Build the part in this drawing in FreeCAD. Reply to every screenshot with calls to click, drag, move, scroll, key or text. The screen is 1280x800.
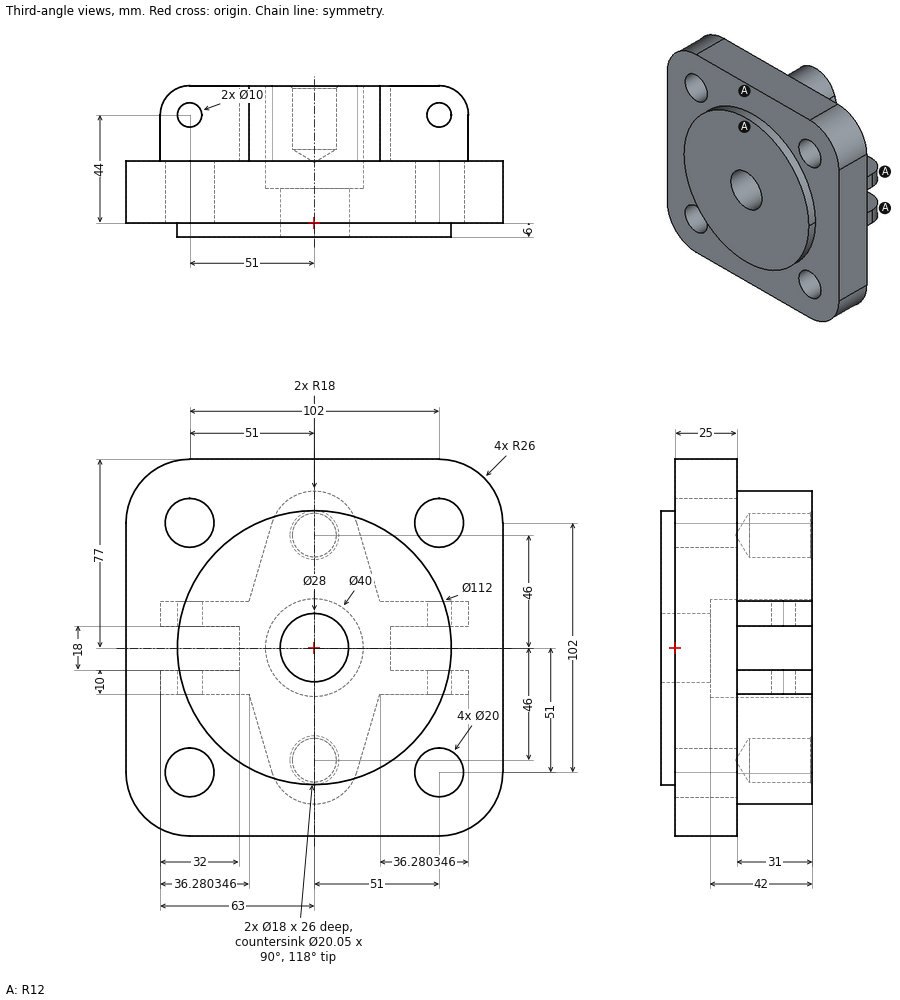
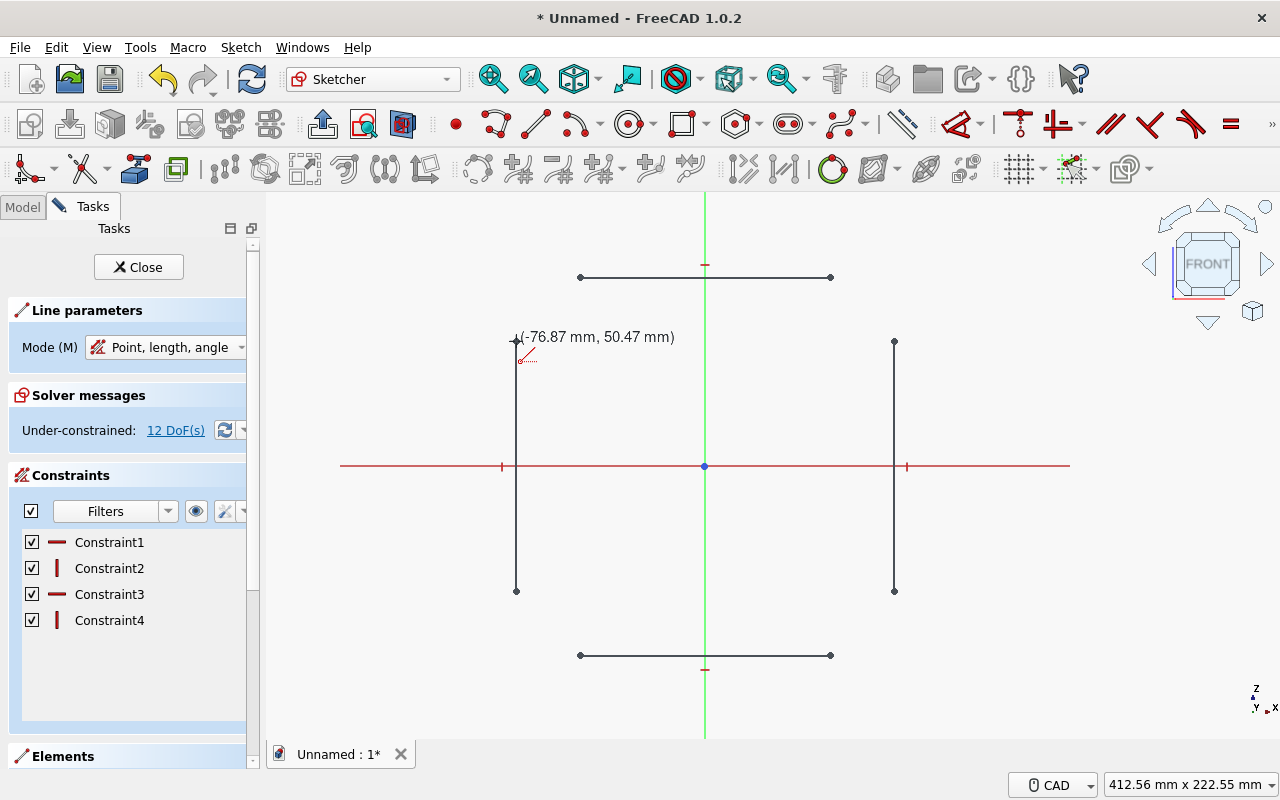
key(g)
key(3)
key(a)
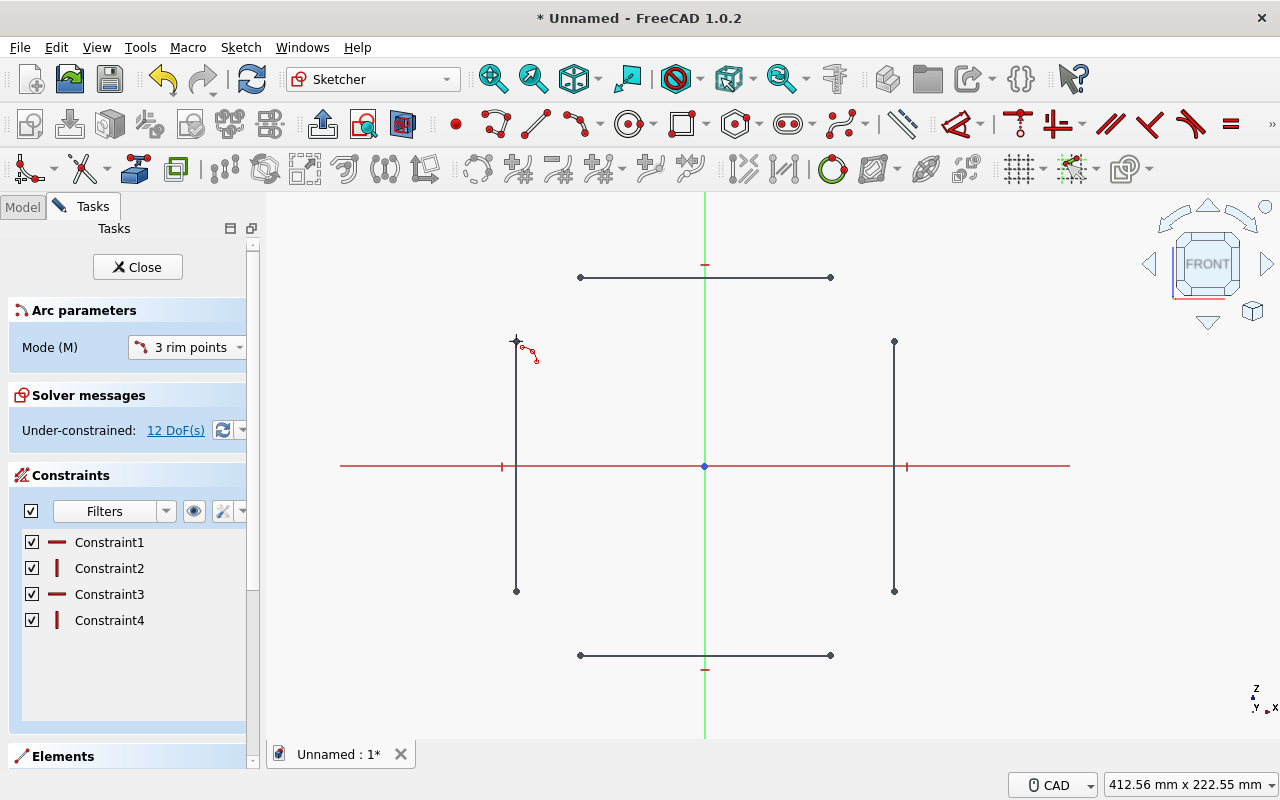
click(830, 278)
click(894, 342)
click(875, 296)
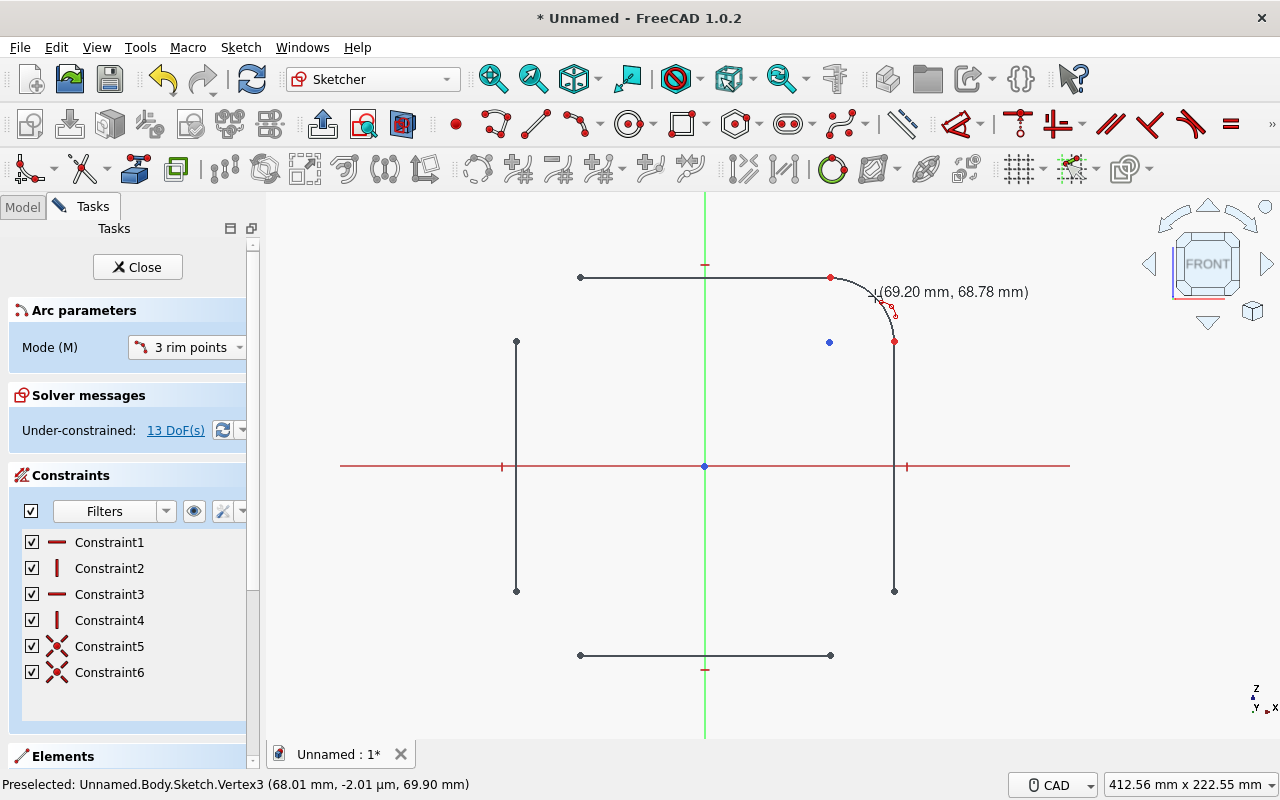
click(894, 592)
click(830, 656)
click(875, 637)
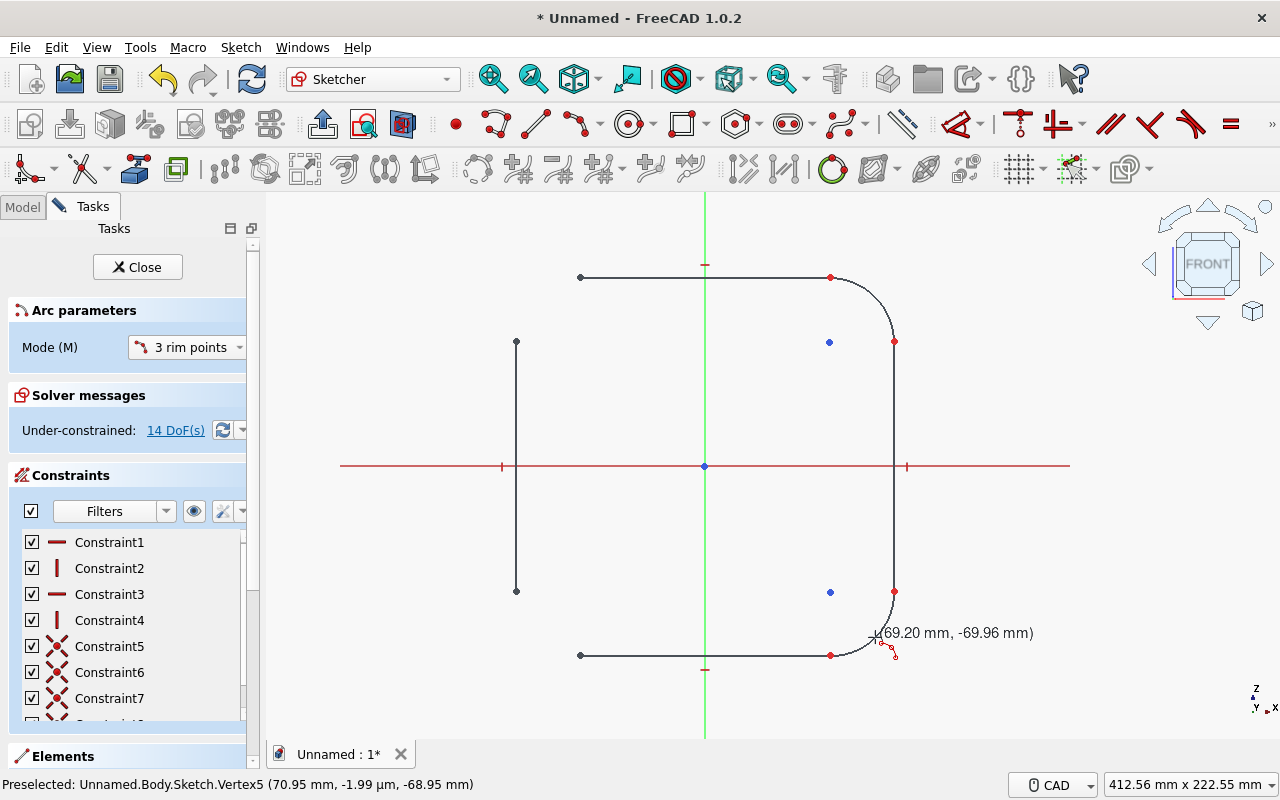
click(580, 656)
click(516, 592)
click(534, 637)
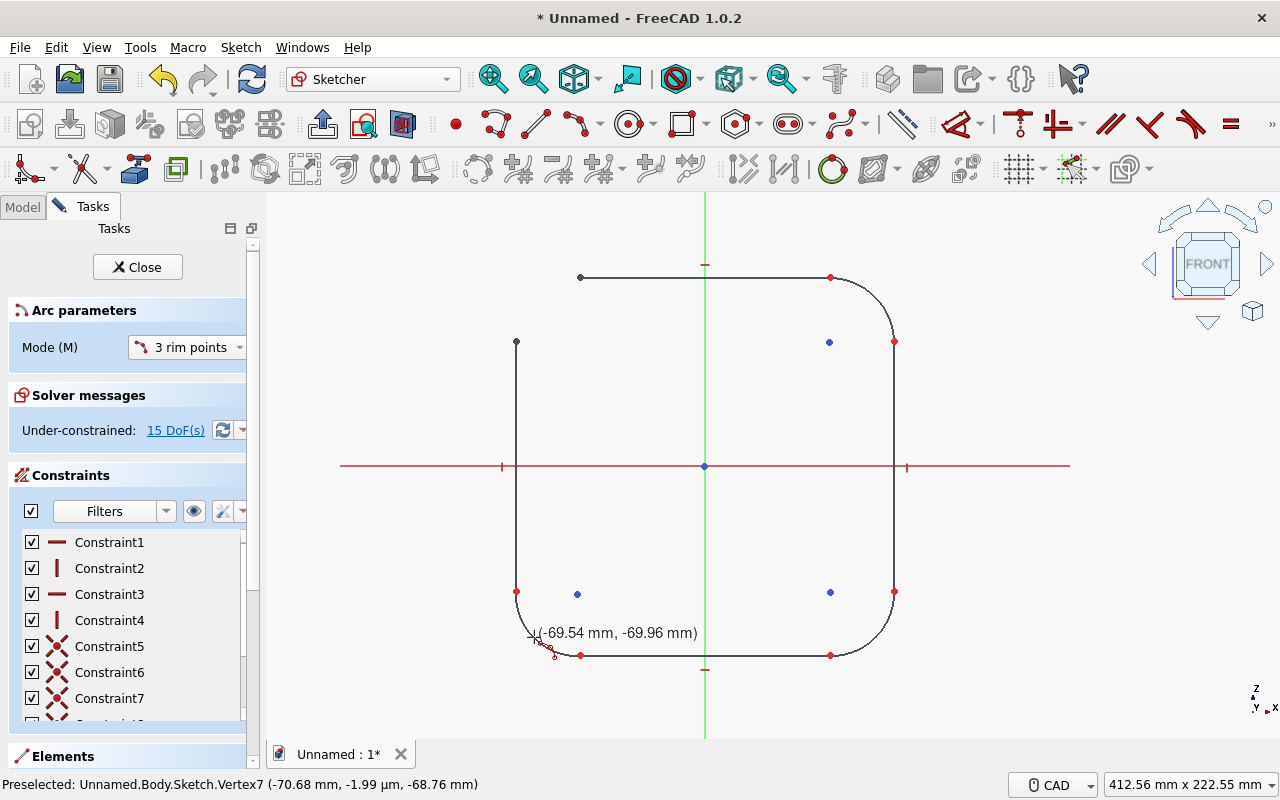
click(516, 342)
click(580, 278)
click(534, 296)
key(Escape)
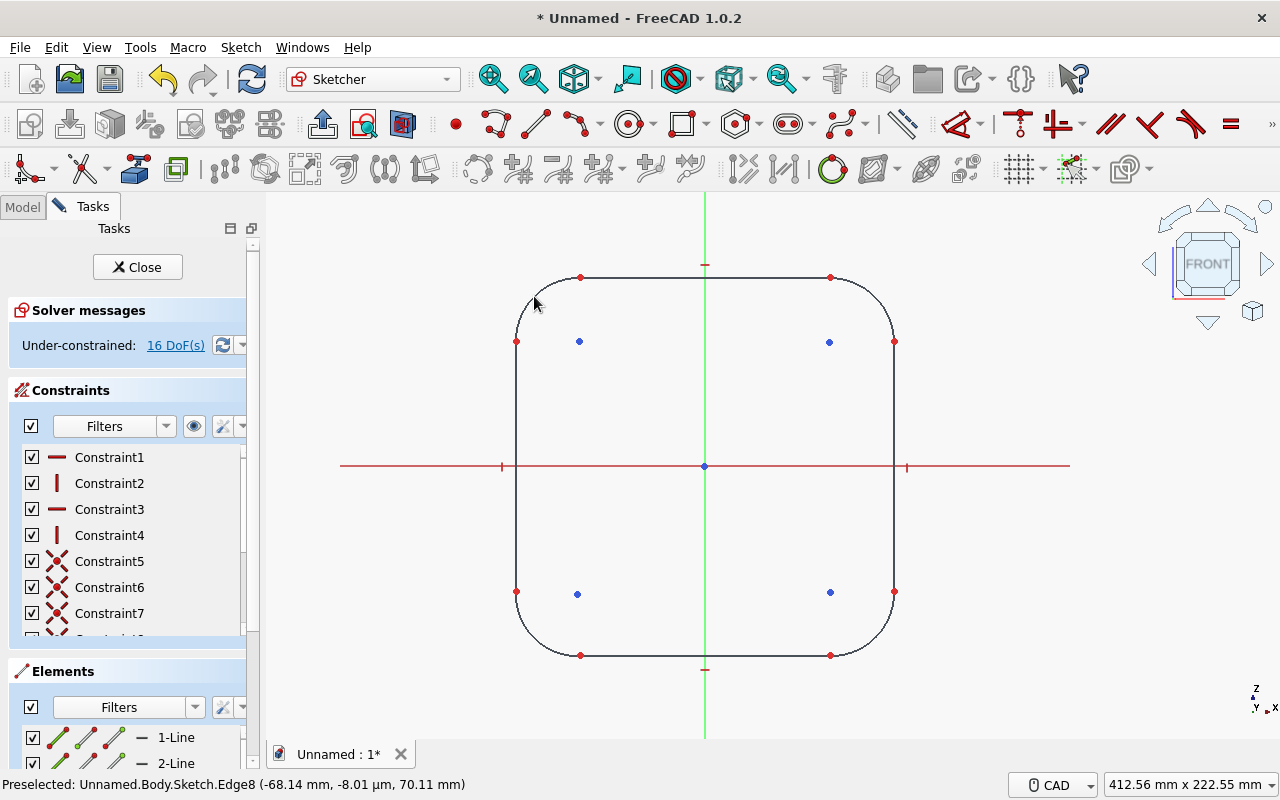
click(655, 278)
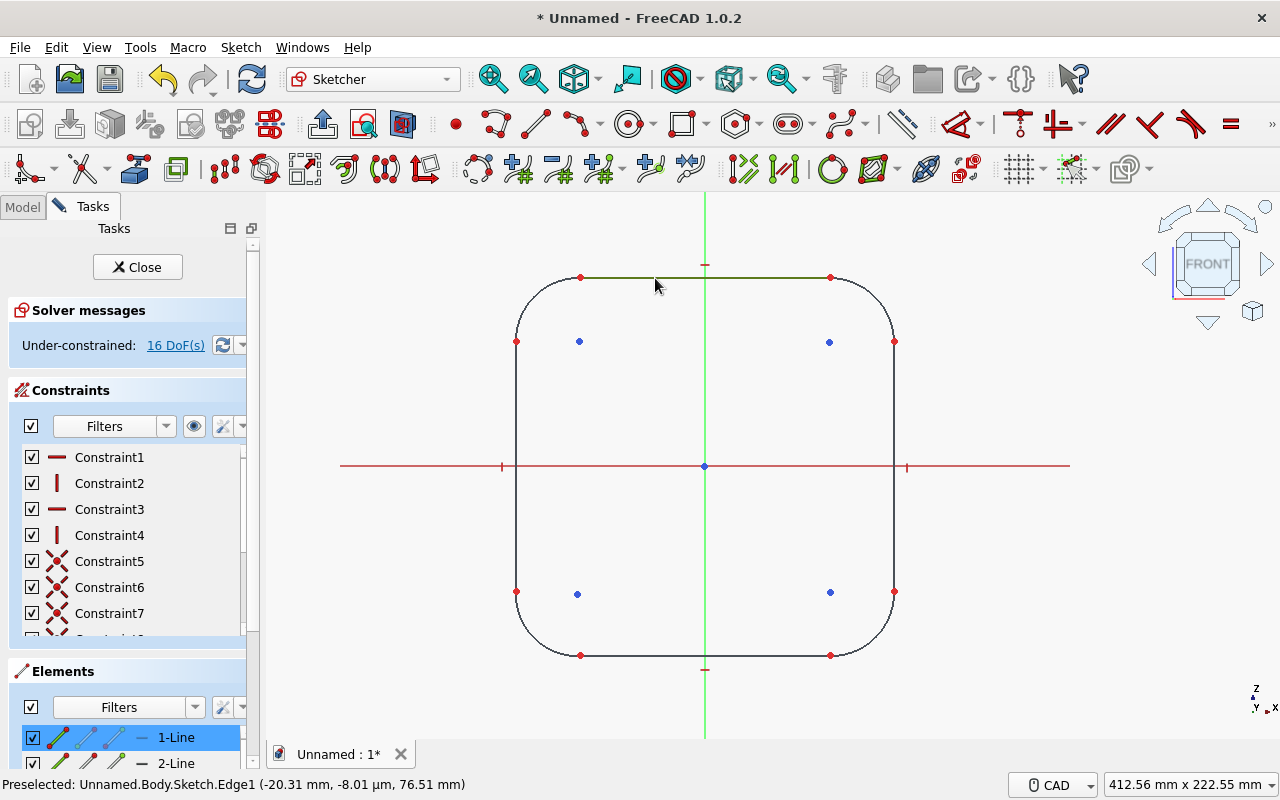
click(887, 313)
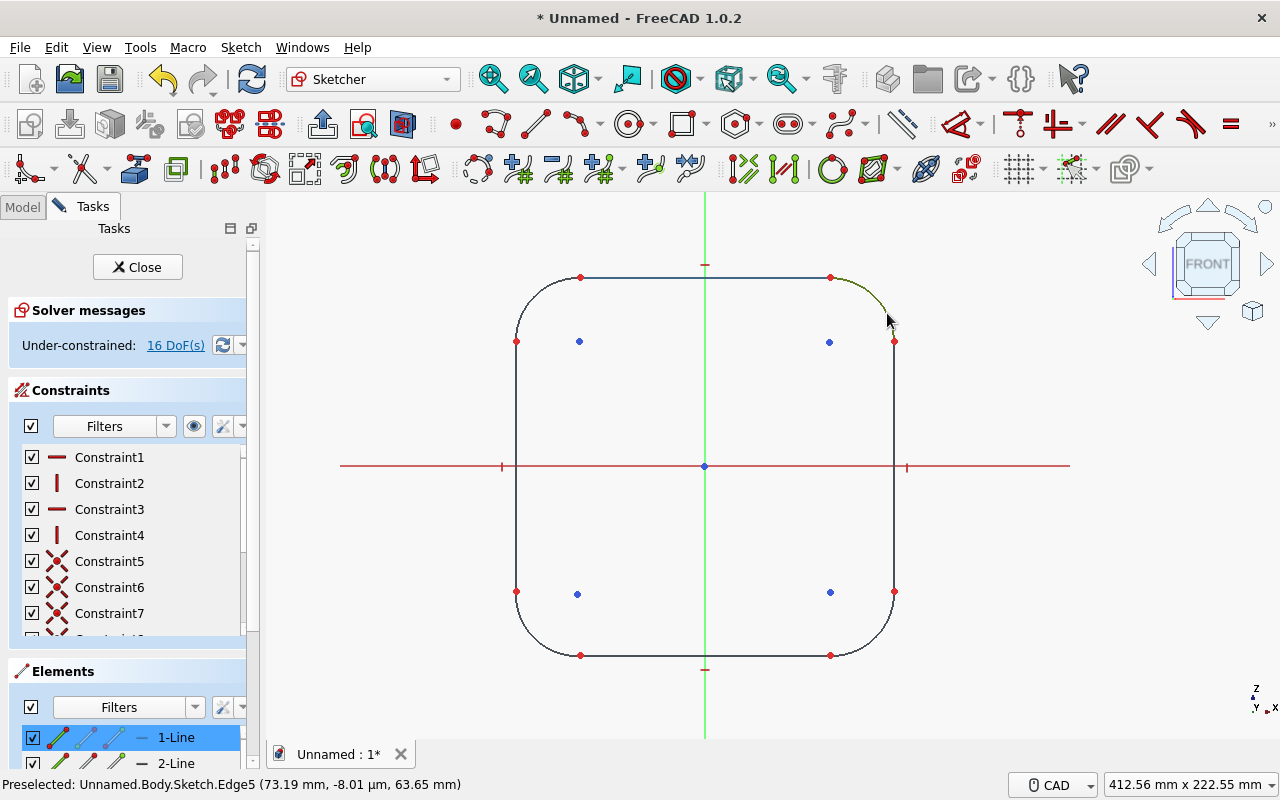
click(1192, 124)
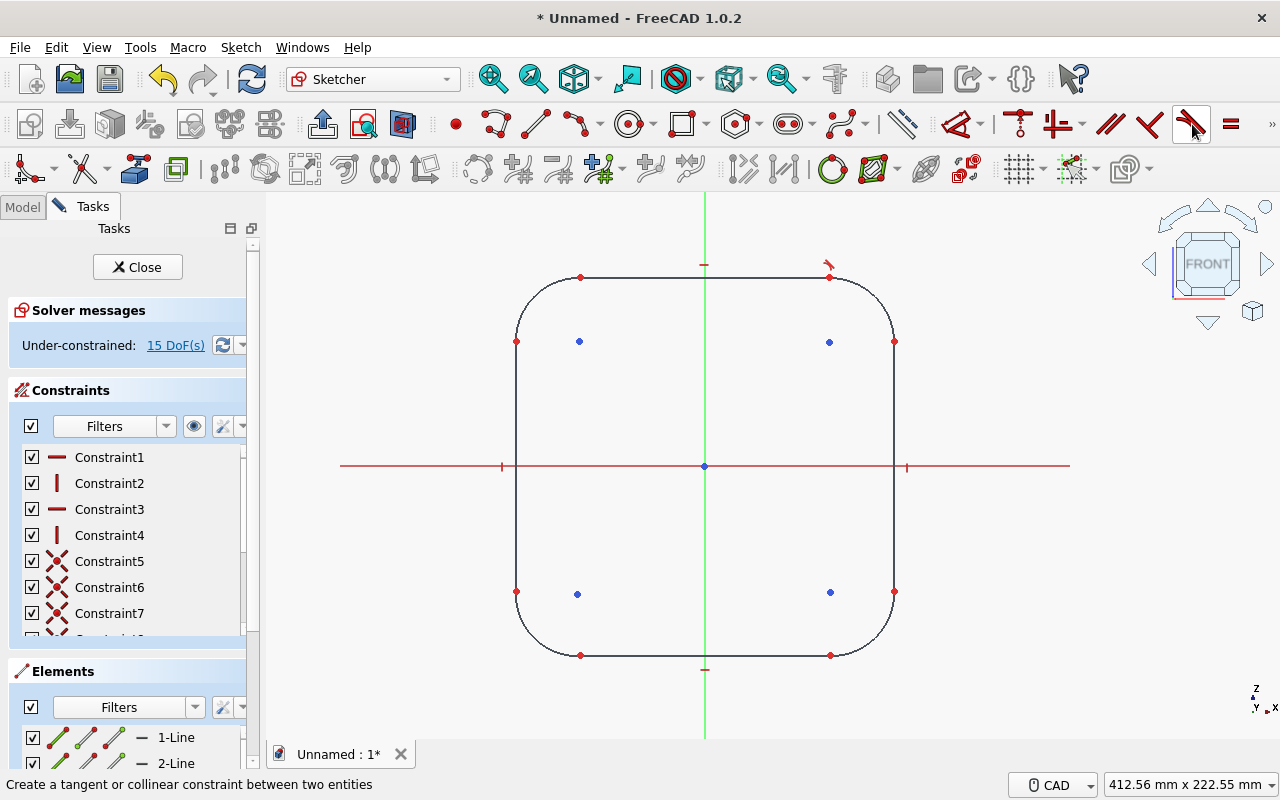
click(655, 278)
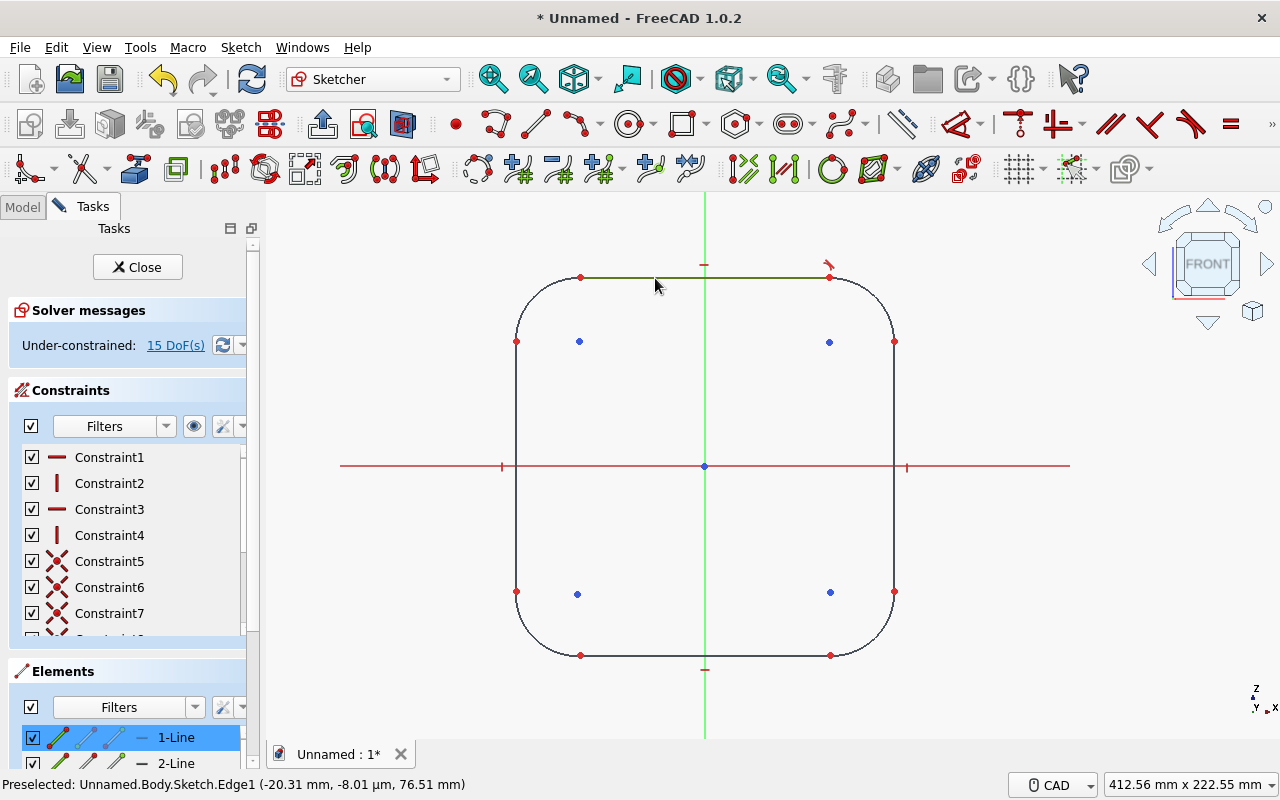
click(551, 285)